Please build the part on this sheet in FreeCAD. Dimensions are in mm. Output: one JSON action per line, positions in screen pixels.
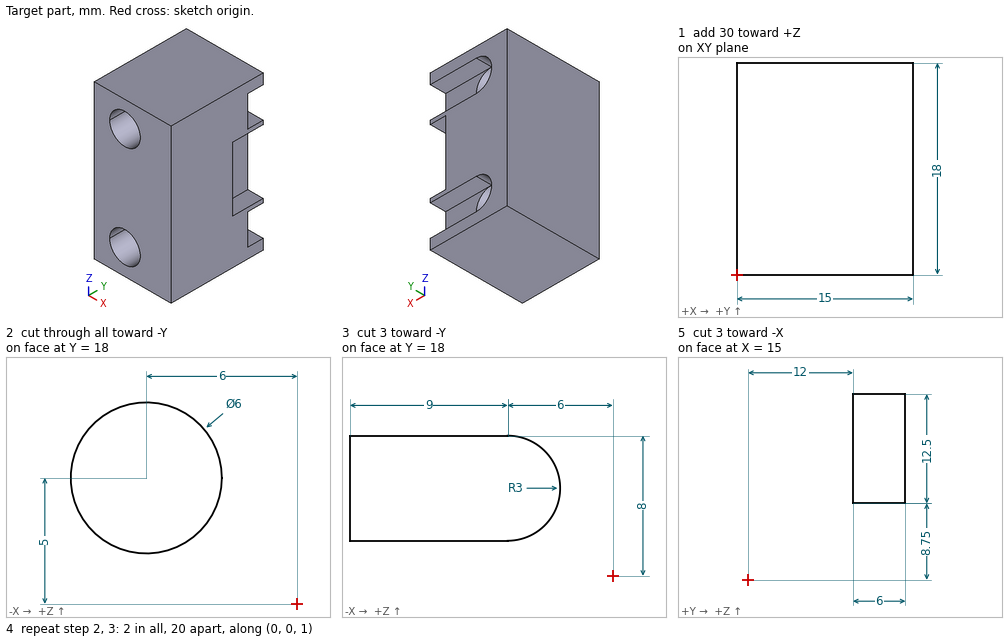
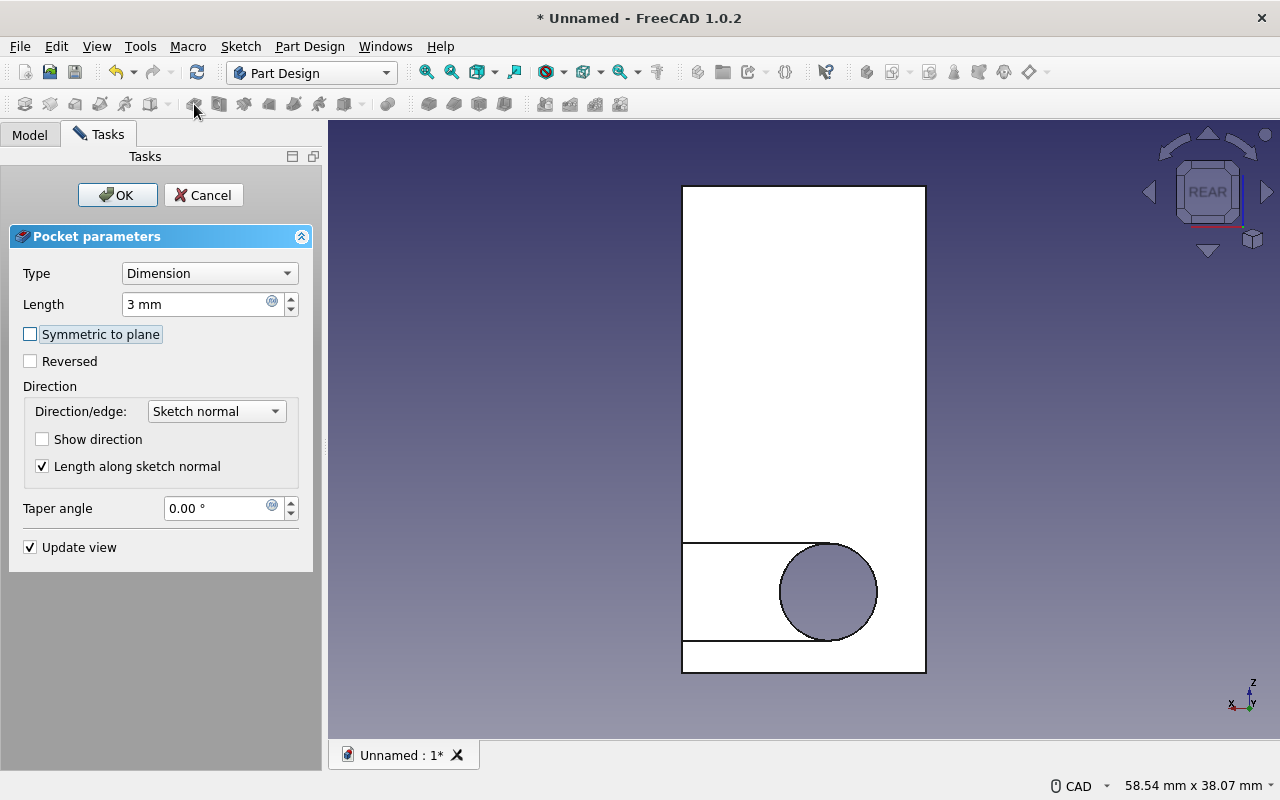
{"action": "left_click", "coordinate": [118, 195]}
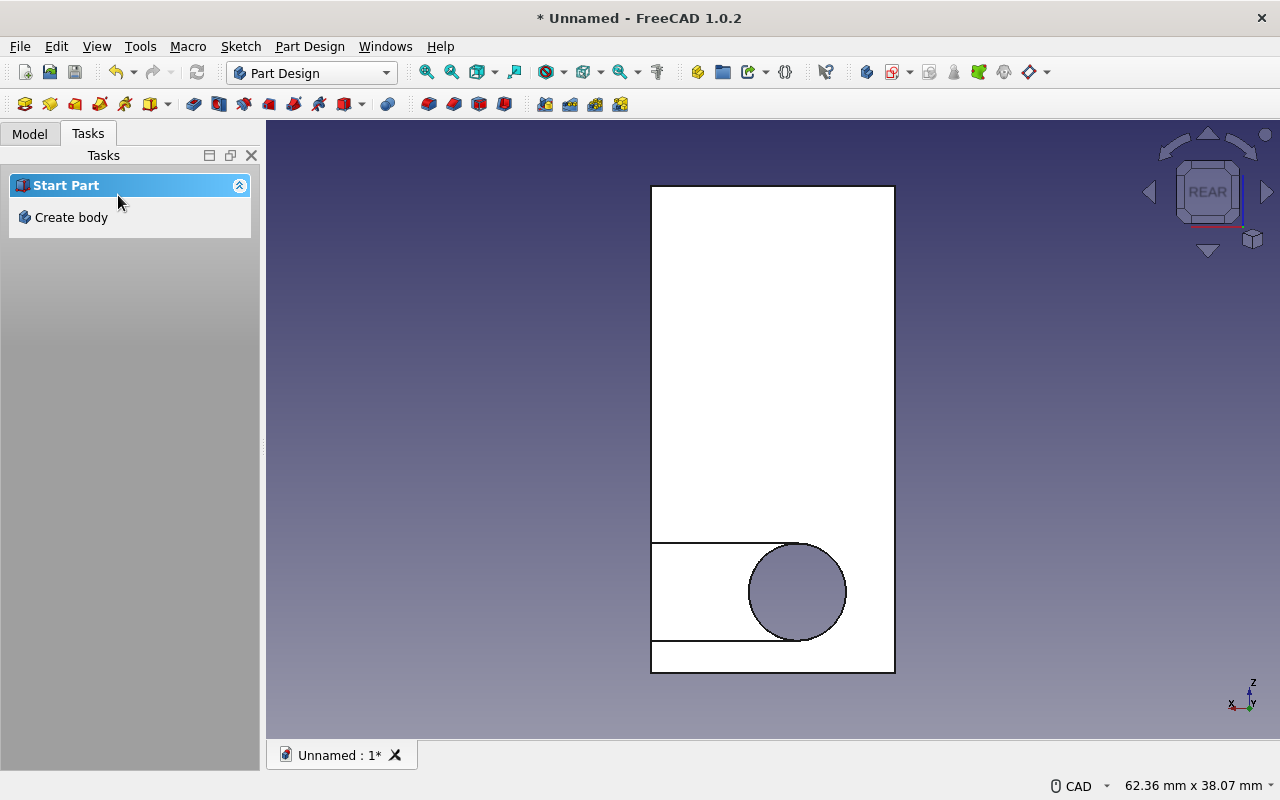
{"action": "left_click", "coordinate": [30, 134]}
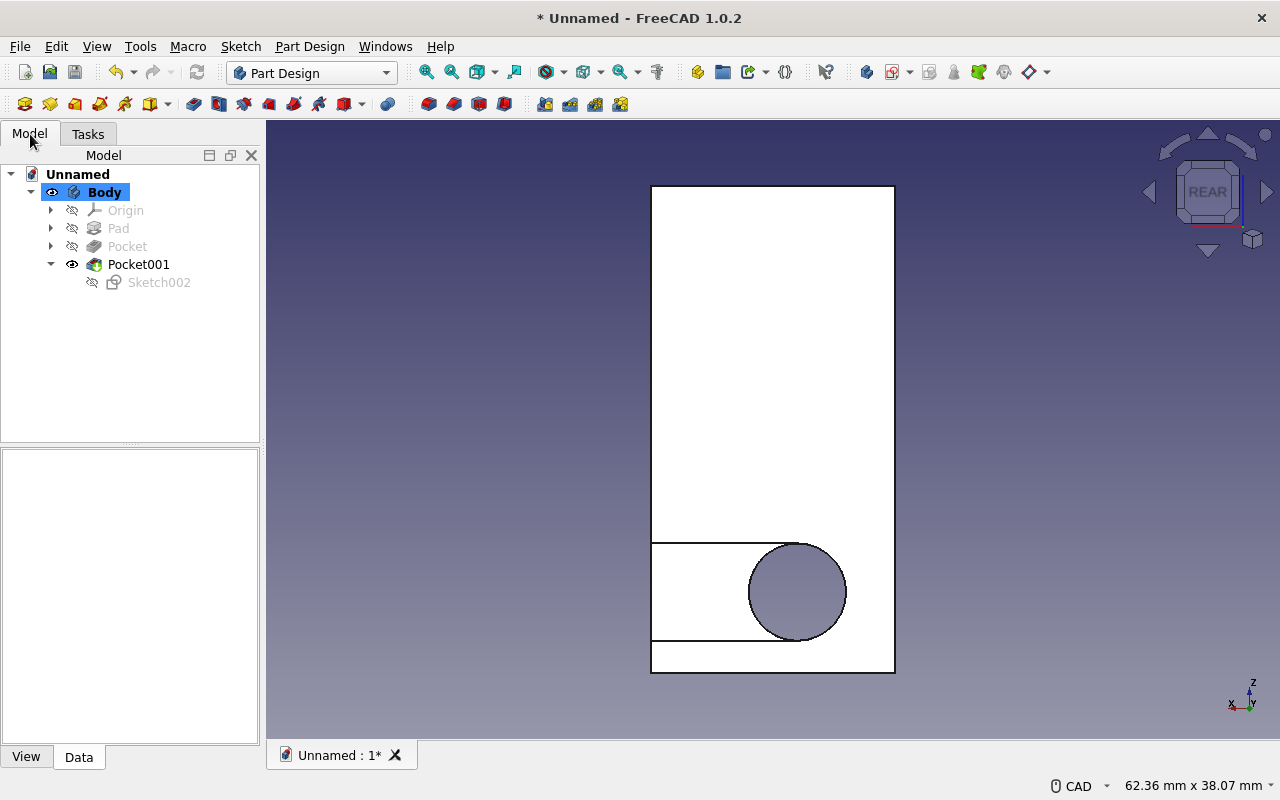
{"action": "left_click", "coordinate": [117, 246]}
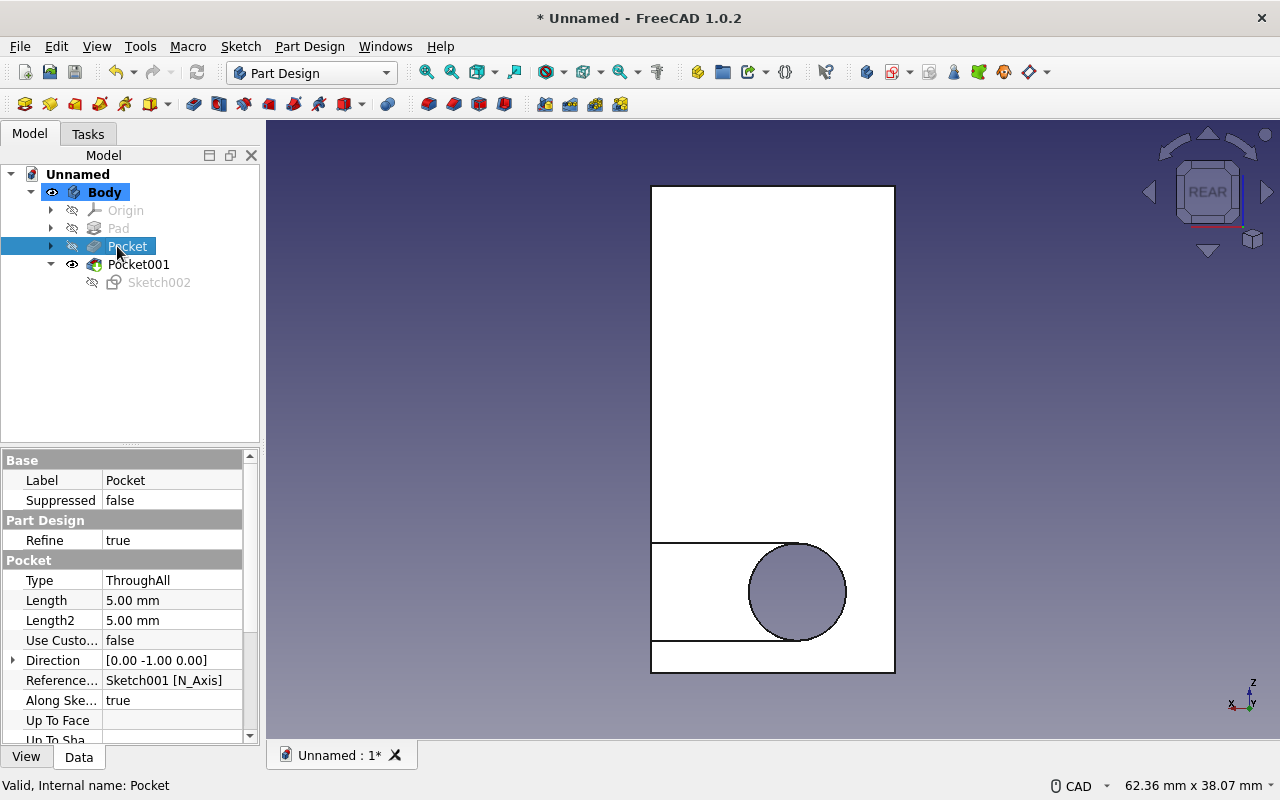
{"action": "left_click", "coordinate": [117, 264], "text": "ctrl"}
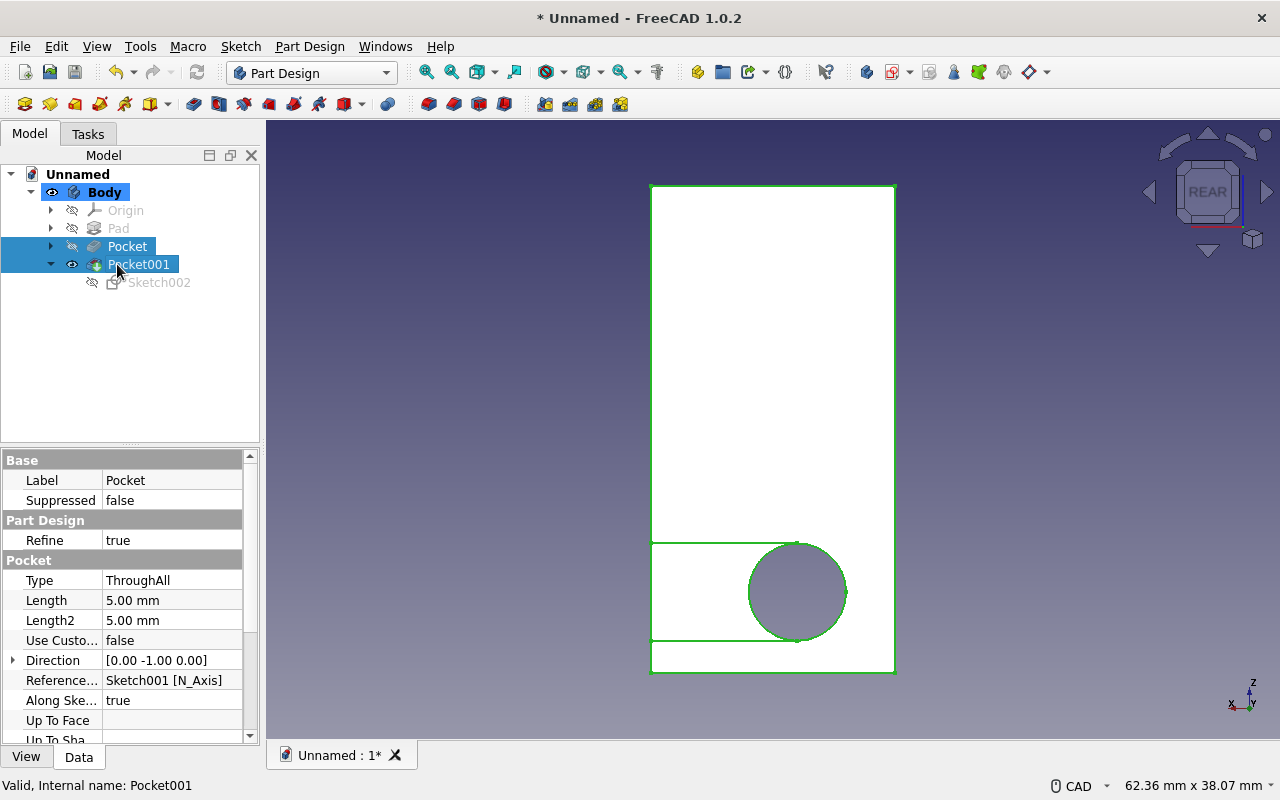
{"action": "left_click", "coordinate": [570, 104]}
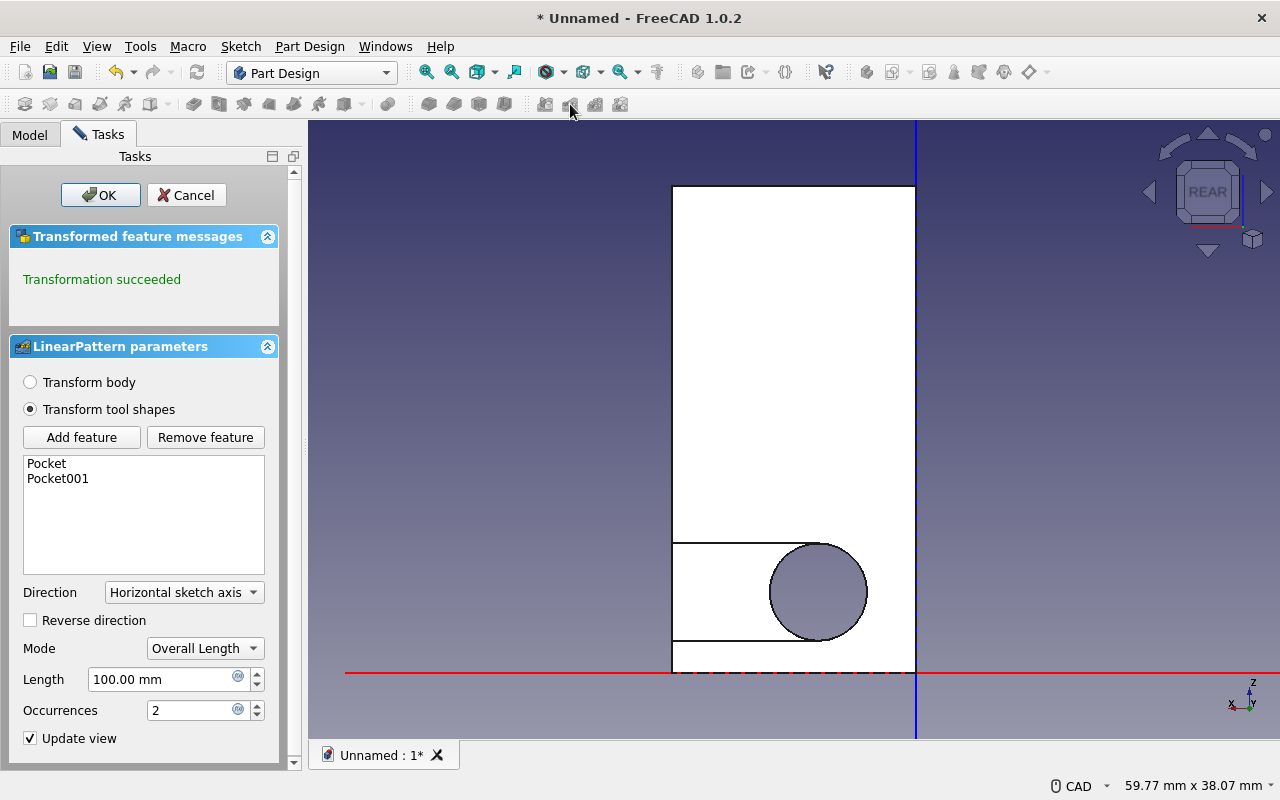
{"action": "left_click", "coordinate": [185, 592]}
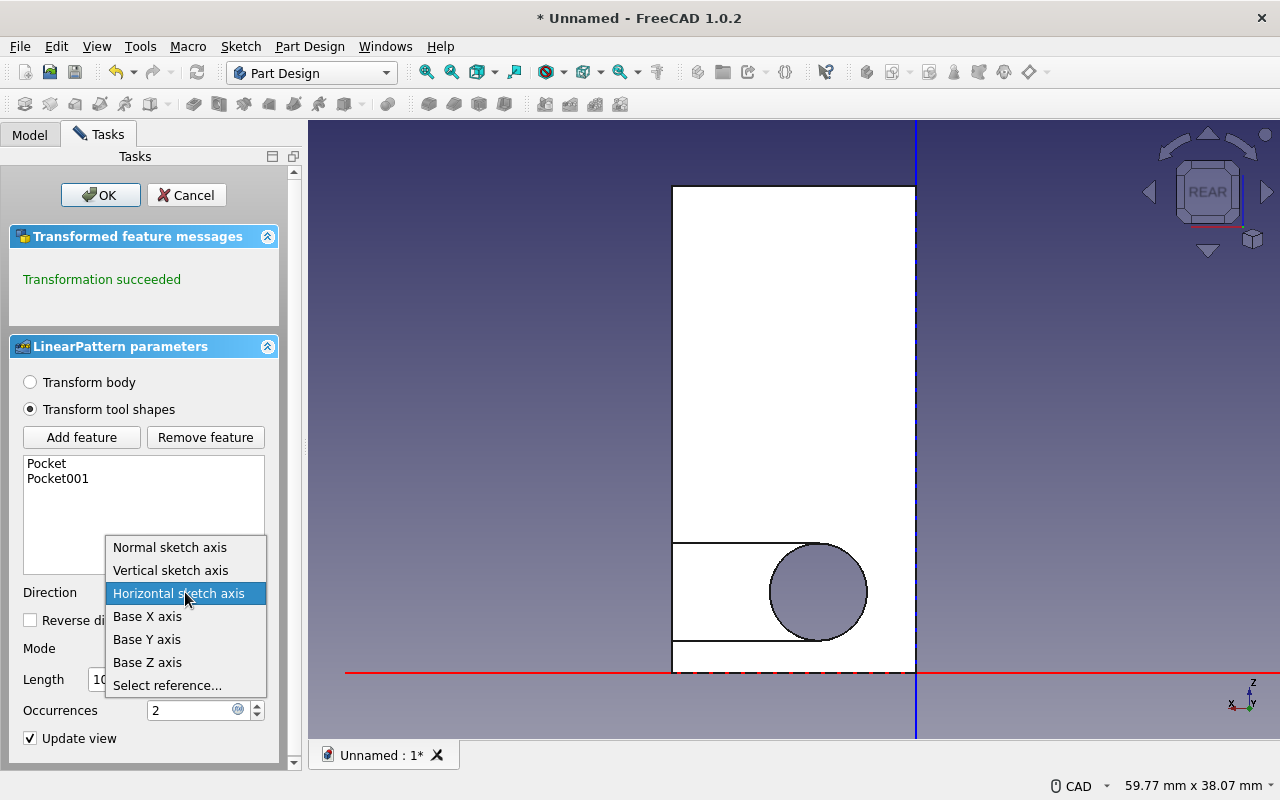
{"action": "left_click", "coordinate": [184, 662]}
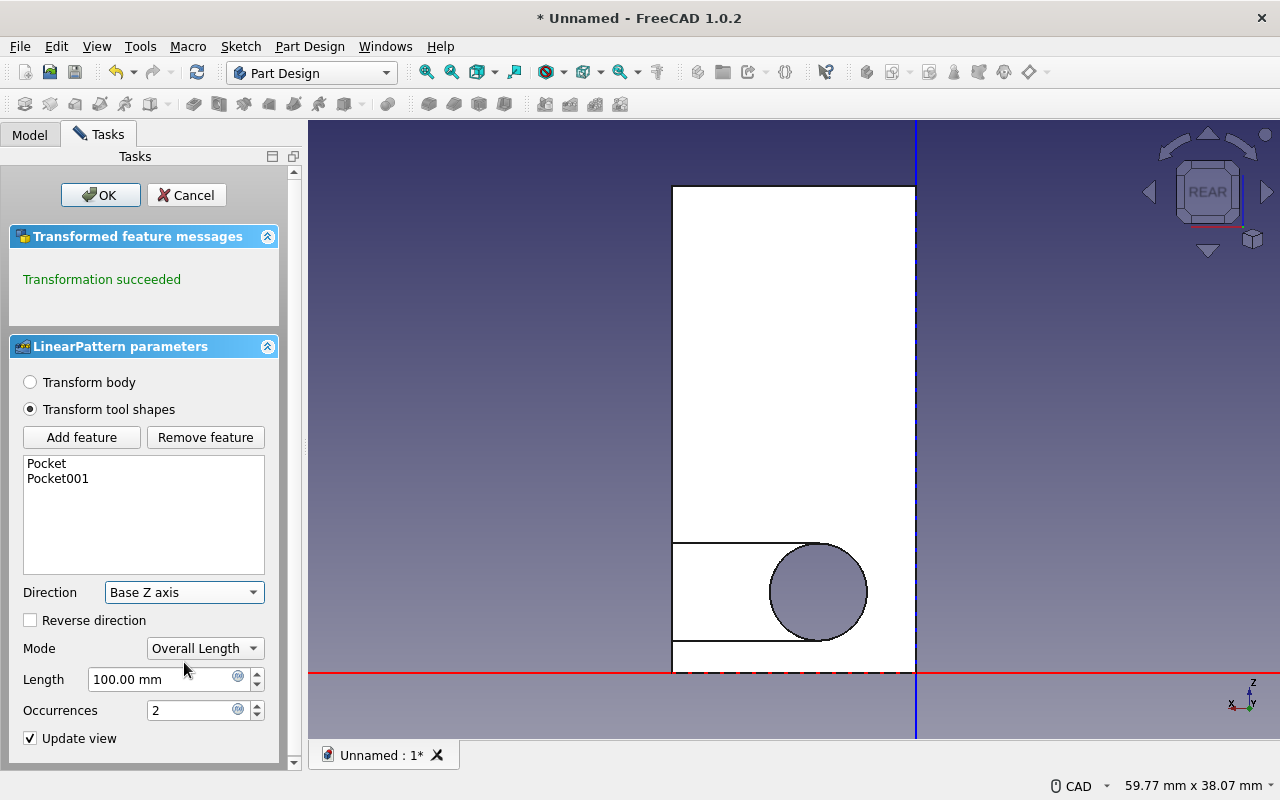
{"action": "left_click", "coordinate": [206, 648]}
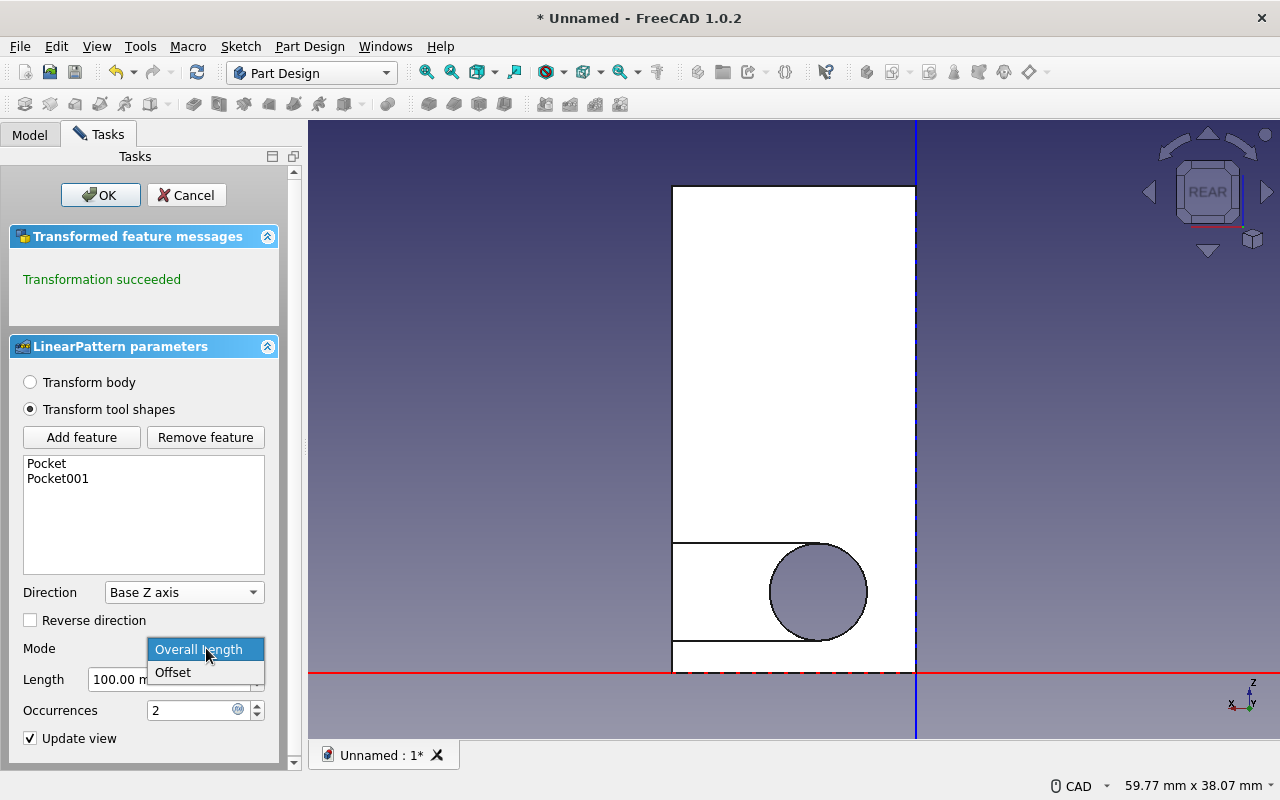
{"action": "left_click", "coordinate": [204, 672]}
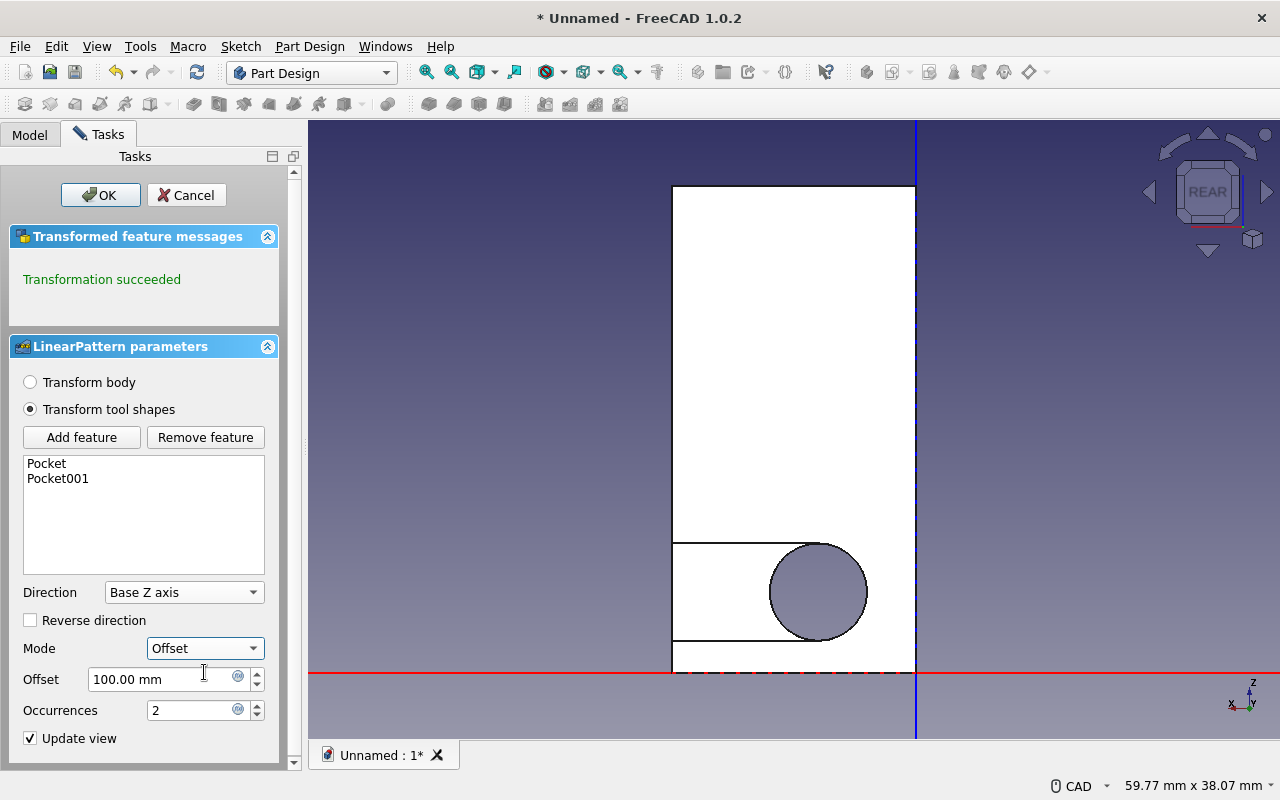
{"action": "triple_click", "coordinate": [170, 680]}